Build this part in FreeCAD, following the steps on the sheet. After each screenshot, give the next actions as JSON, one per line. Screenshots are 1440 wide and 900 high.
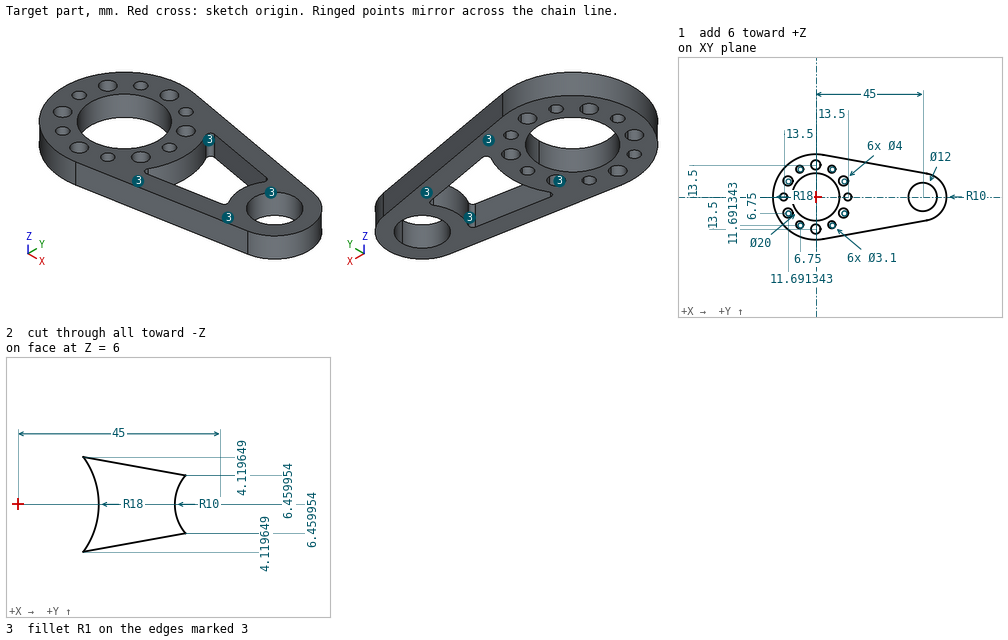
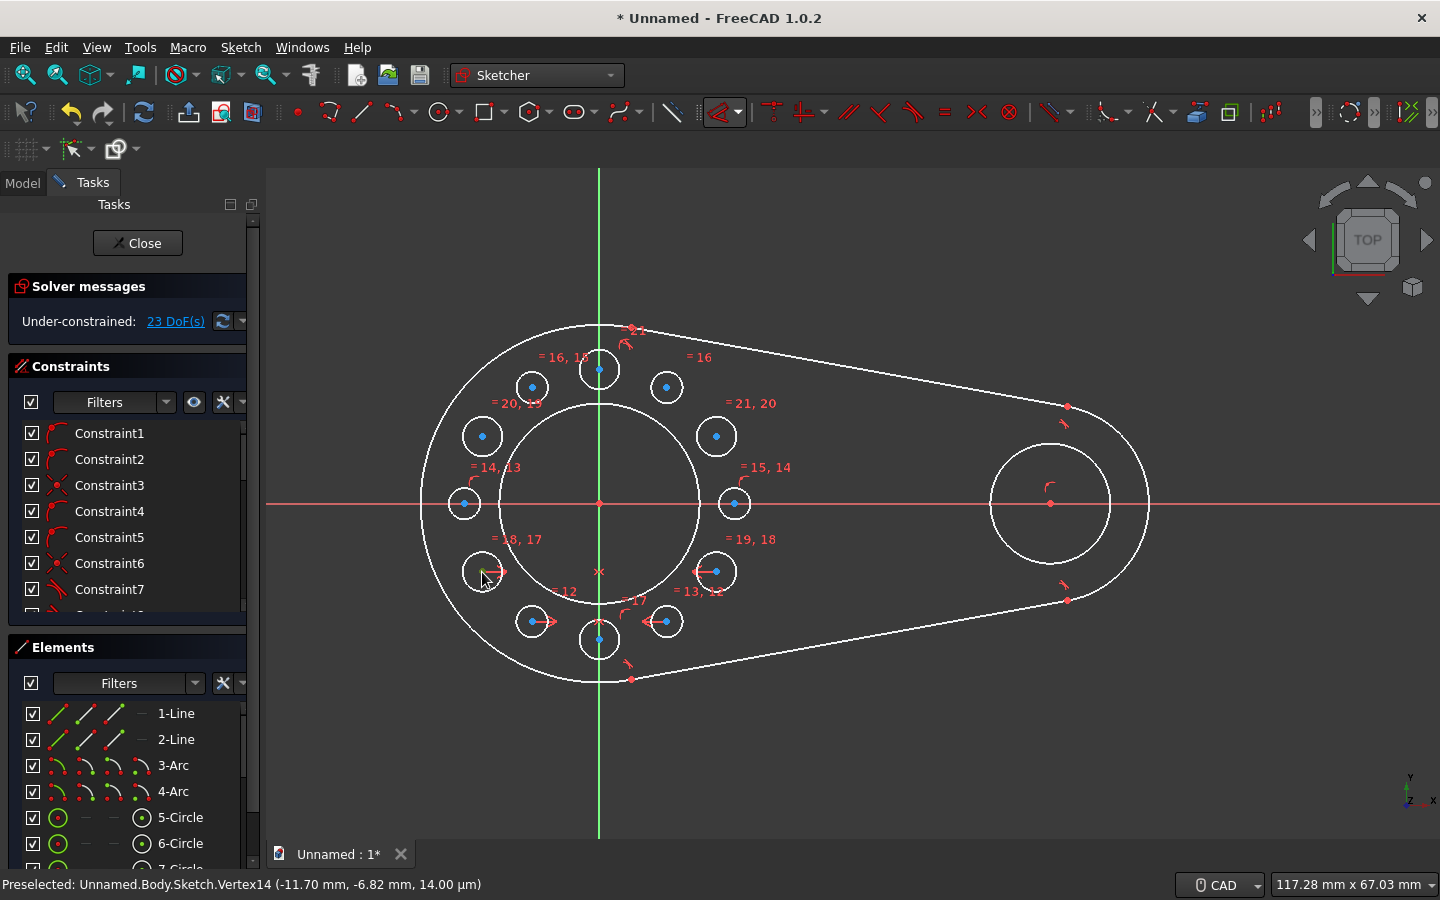
{"action": "left_click", "coordinate": [483, 437]}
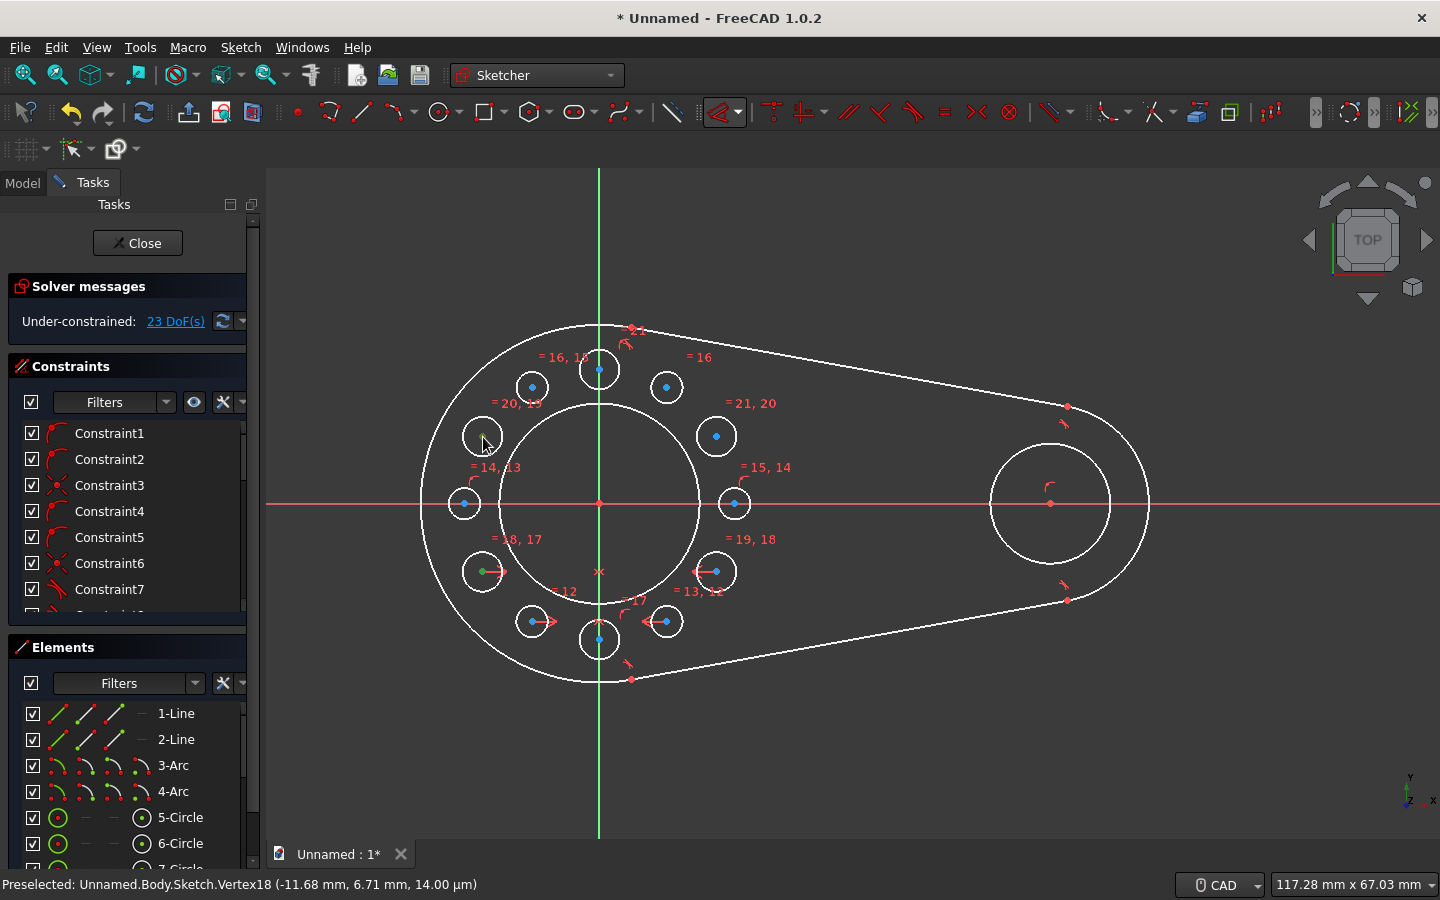
{"action": "left_click", "coordinate": [364, 504]}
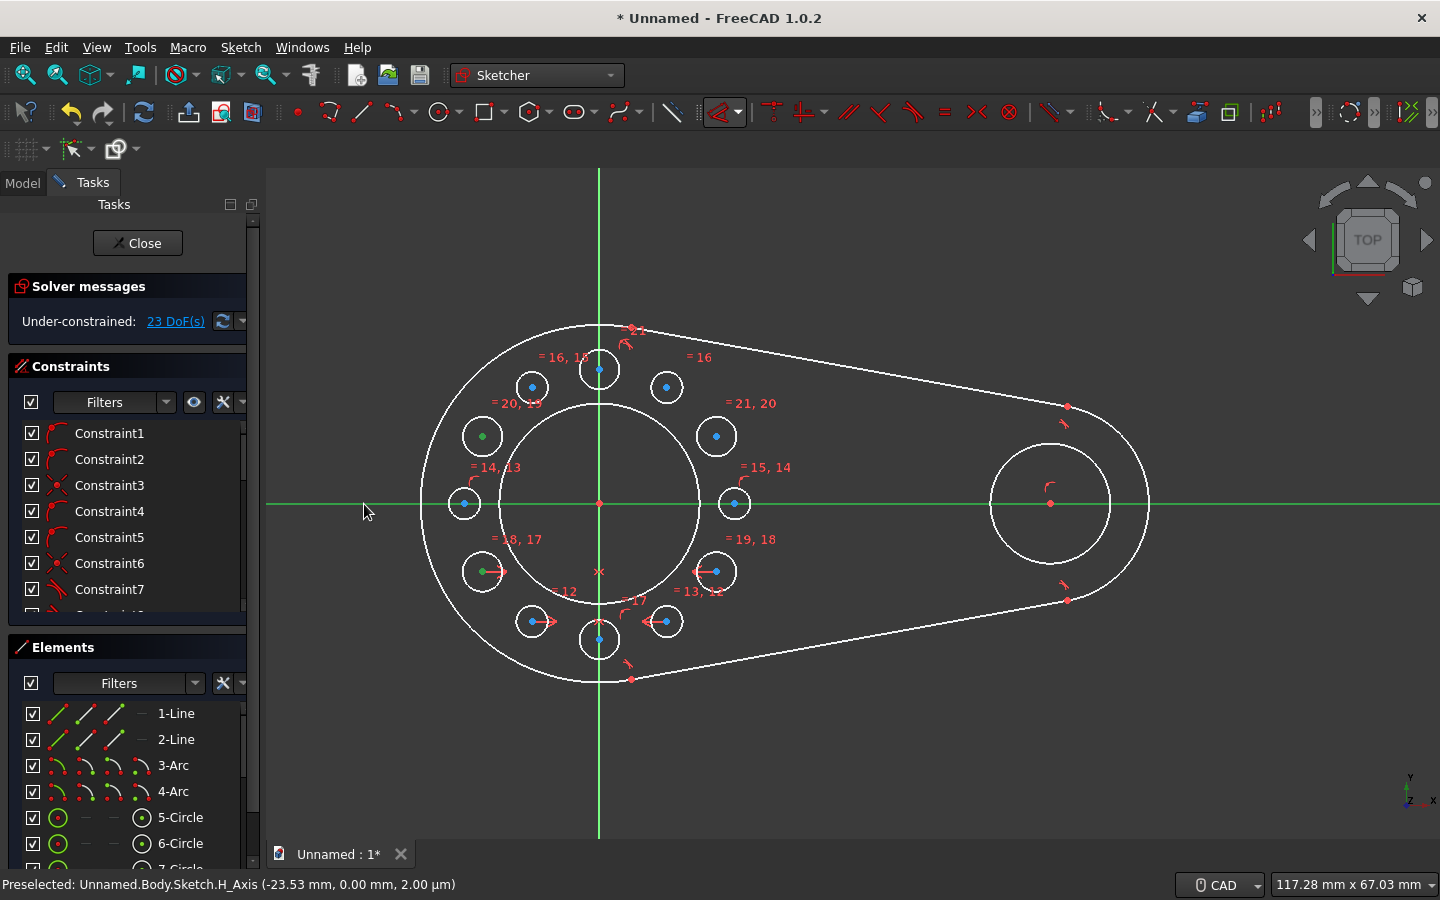
{"action": "key", "text": "s"}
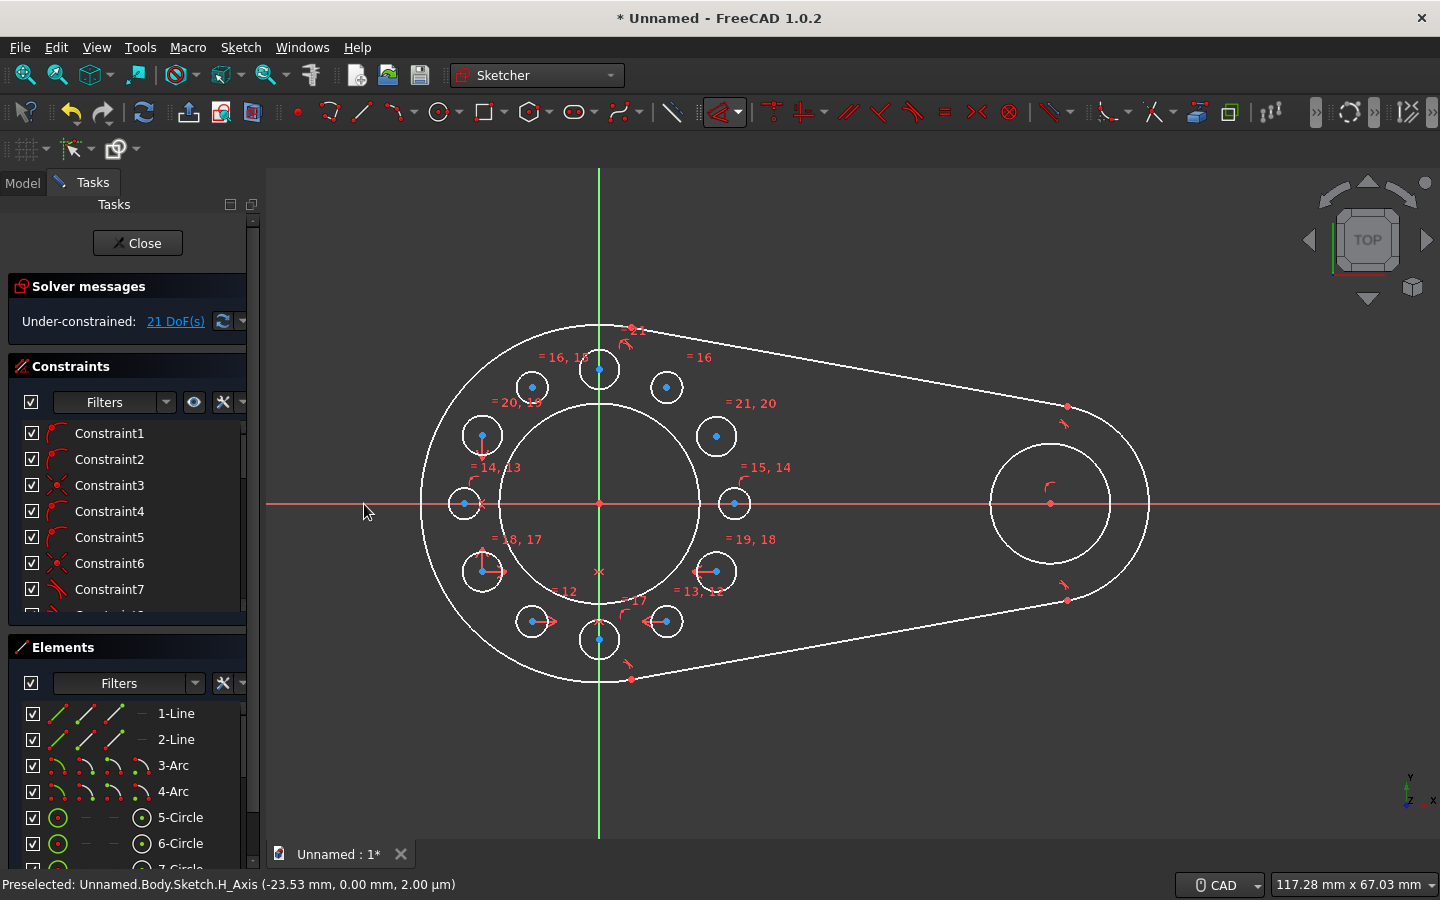
{"action": "left_click", "coordinate": [717, 572]}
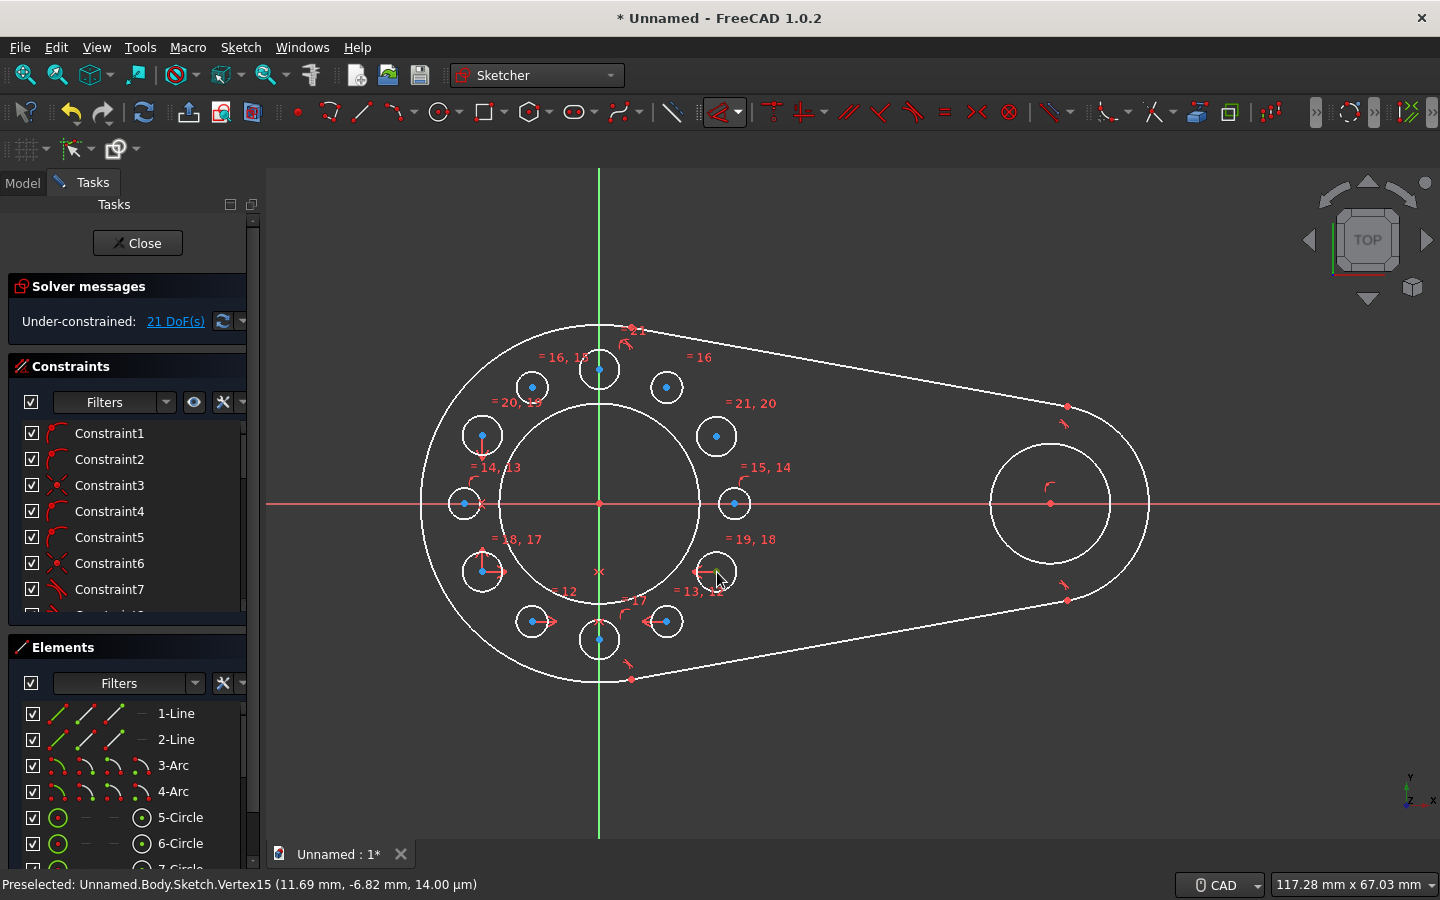
{"action": "left_click", "coordinate": [717, 437]}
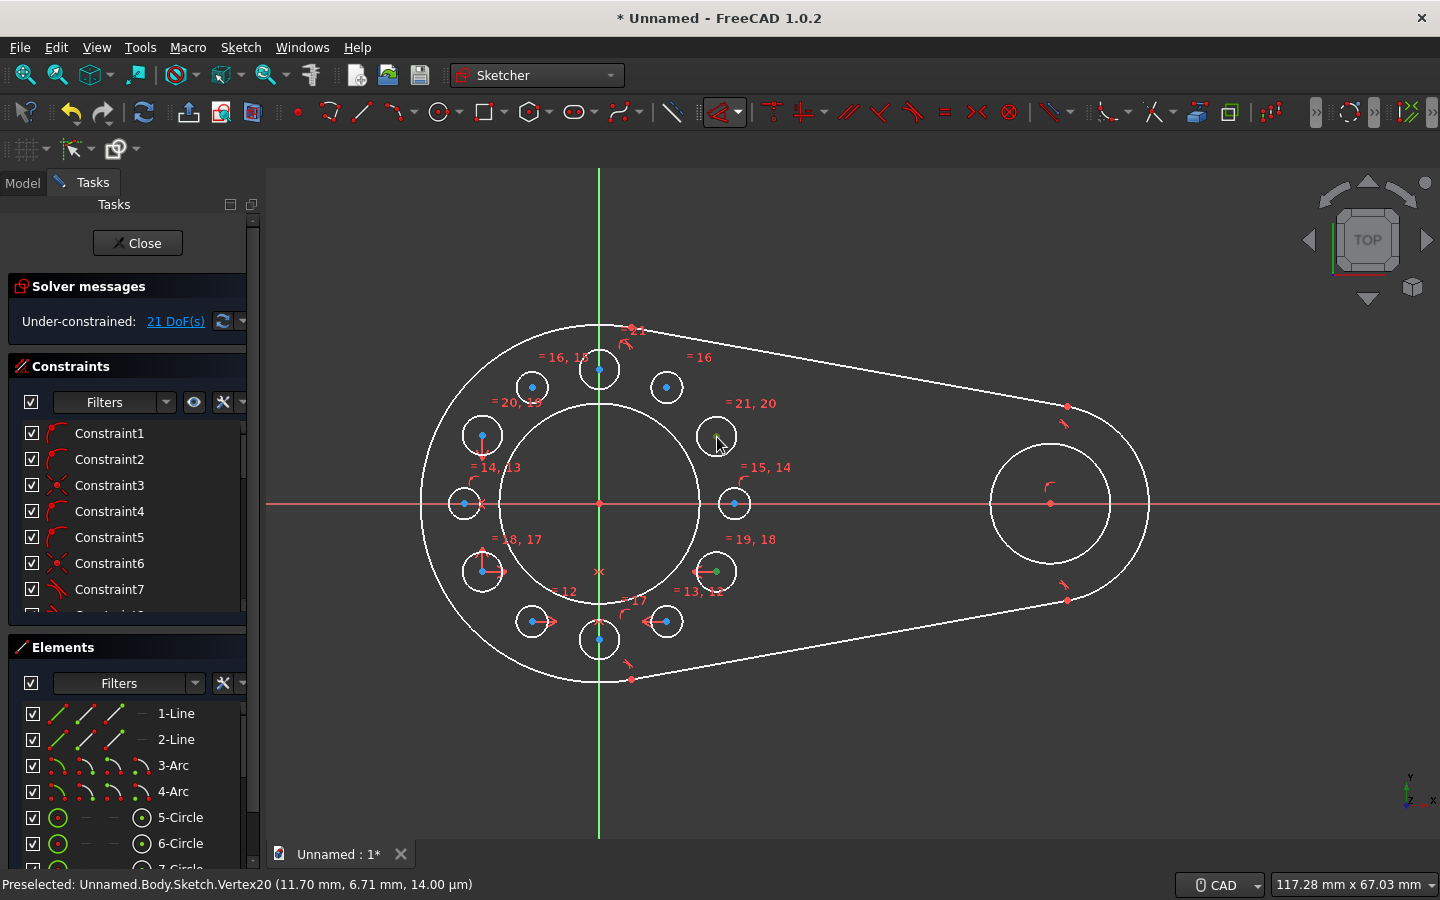
{"action": "left_click", "coordinate": [364, 504]}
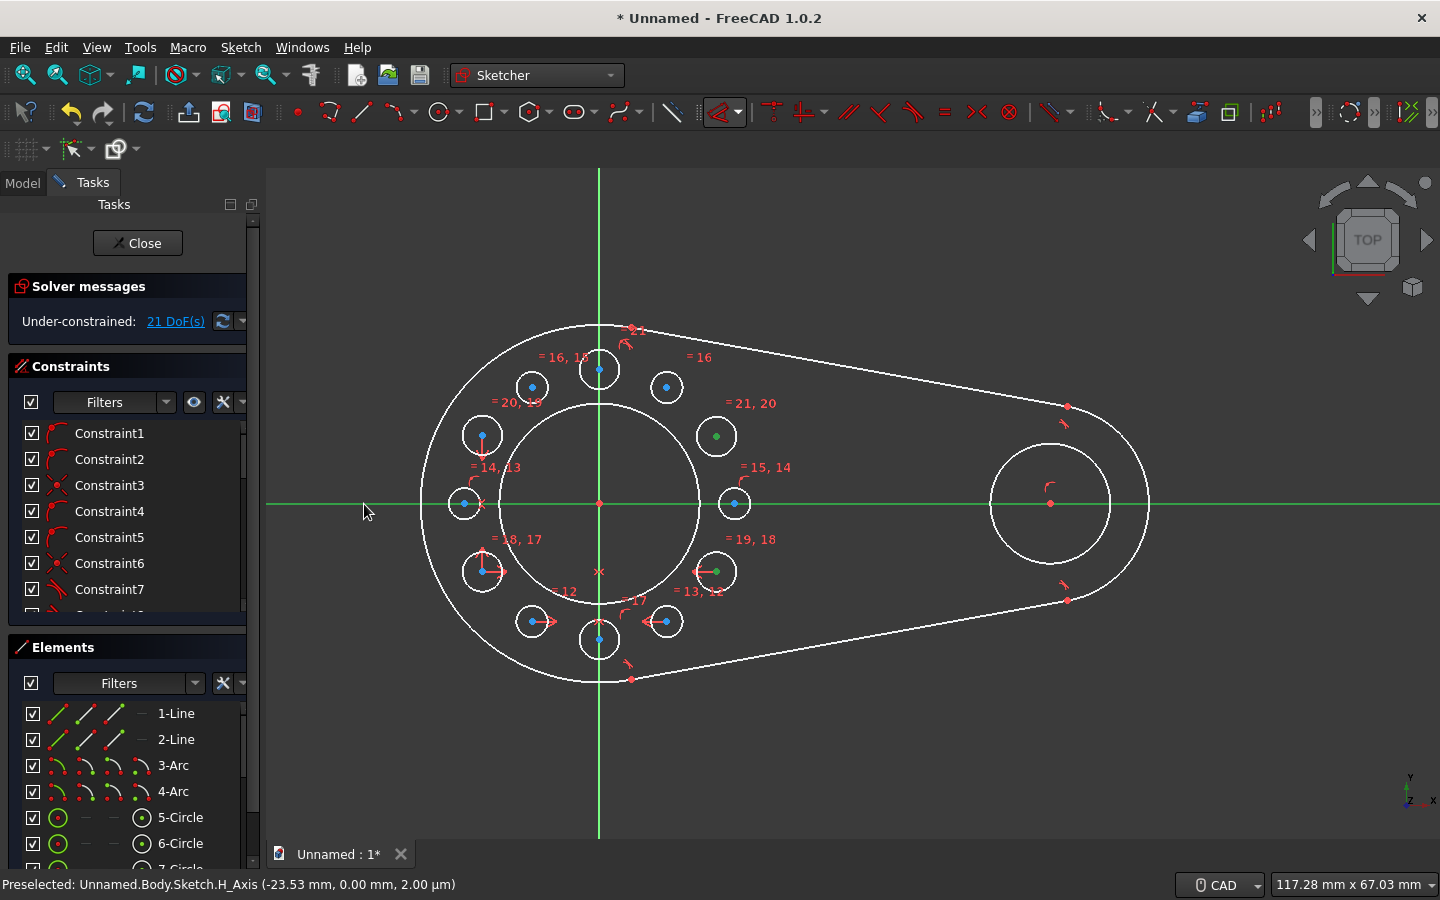
{"action": "left_click", "coordinate": [978, 112]}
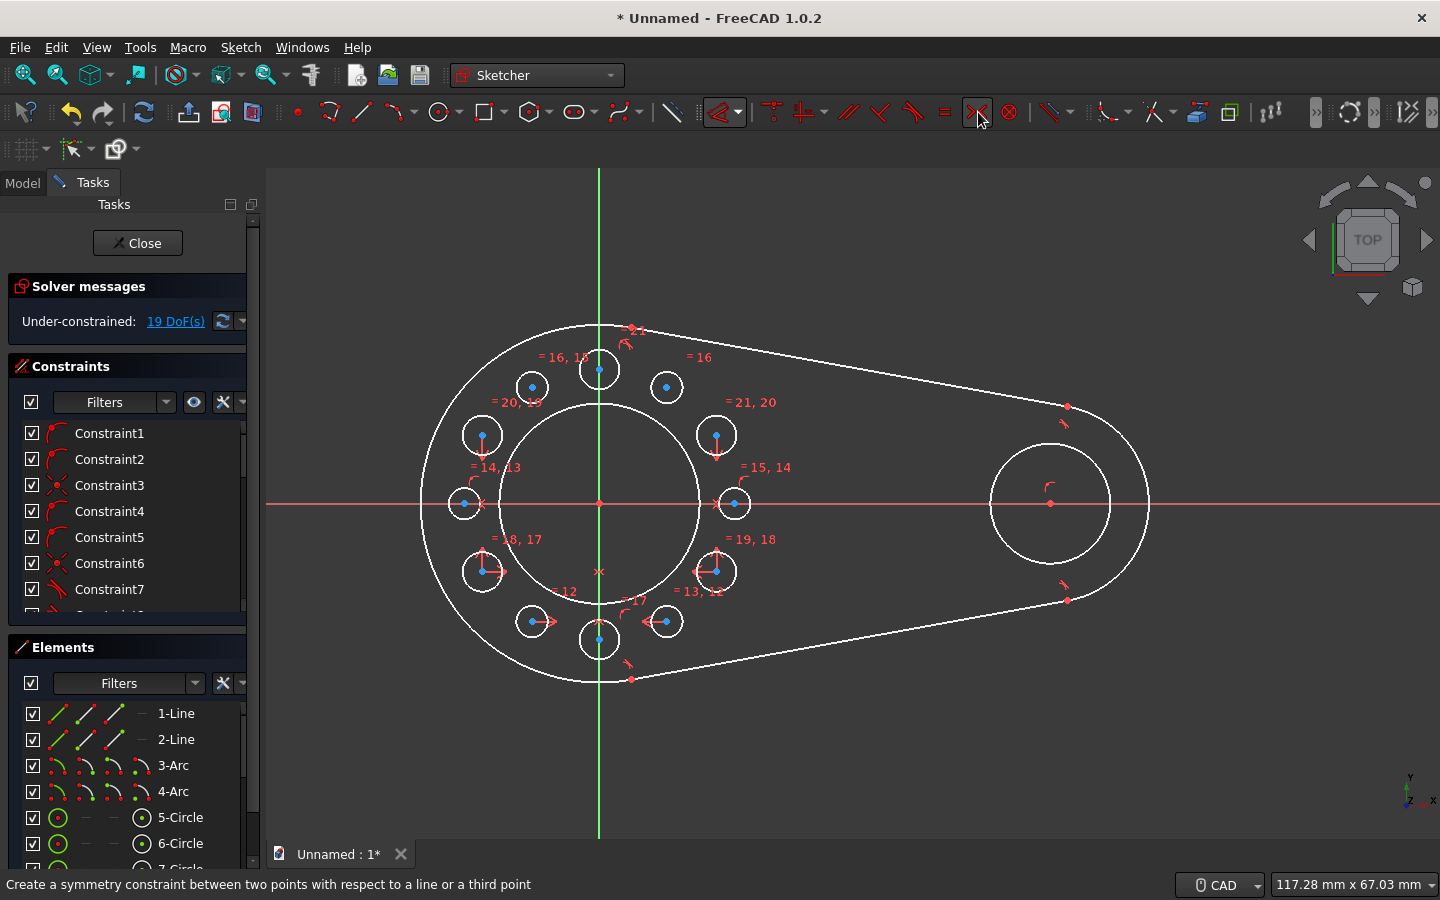
{"action": "left_click", "coordinate": [532, 622]}